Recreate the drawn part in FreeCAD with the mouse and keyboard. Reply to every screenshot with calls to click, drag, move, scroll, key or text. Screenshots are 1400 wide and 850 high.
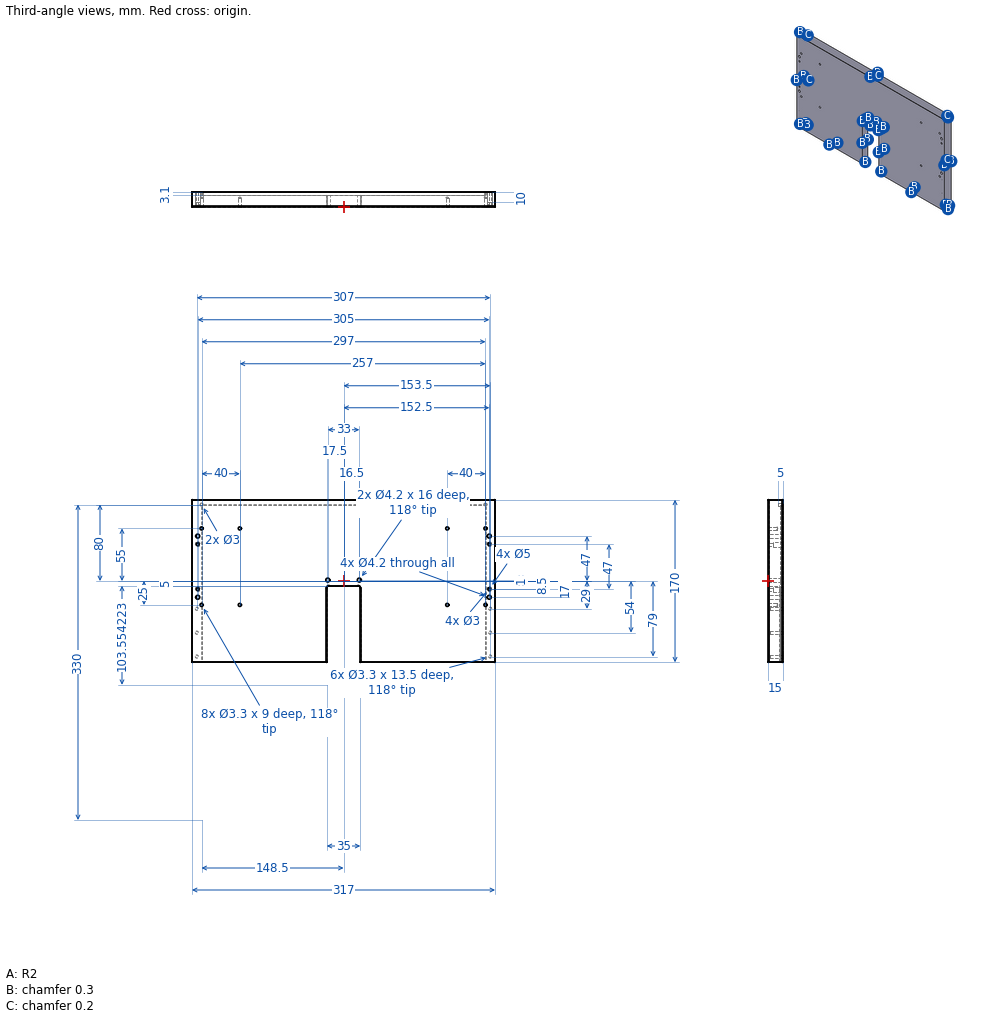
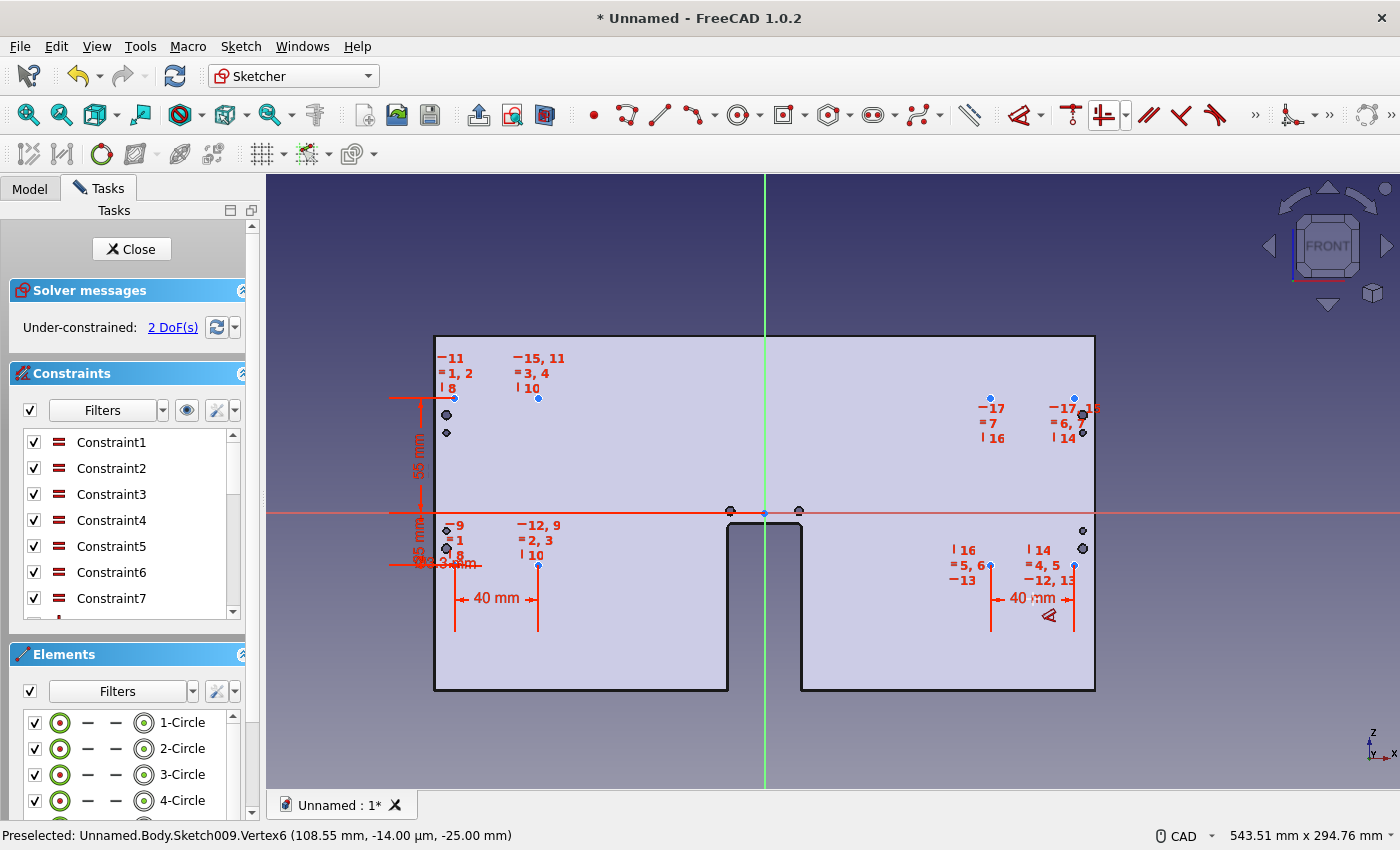
click(538, 565)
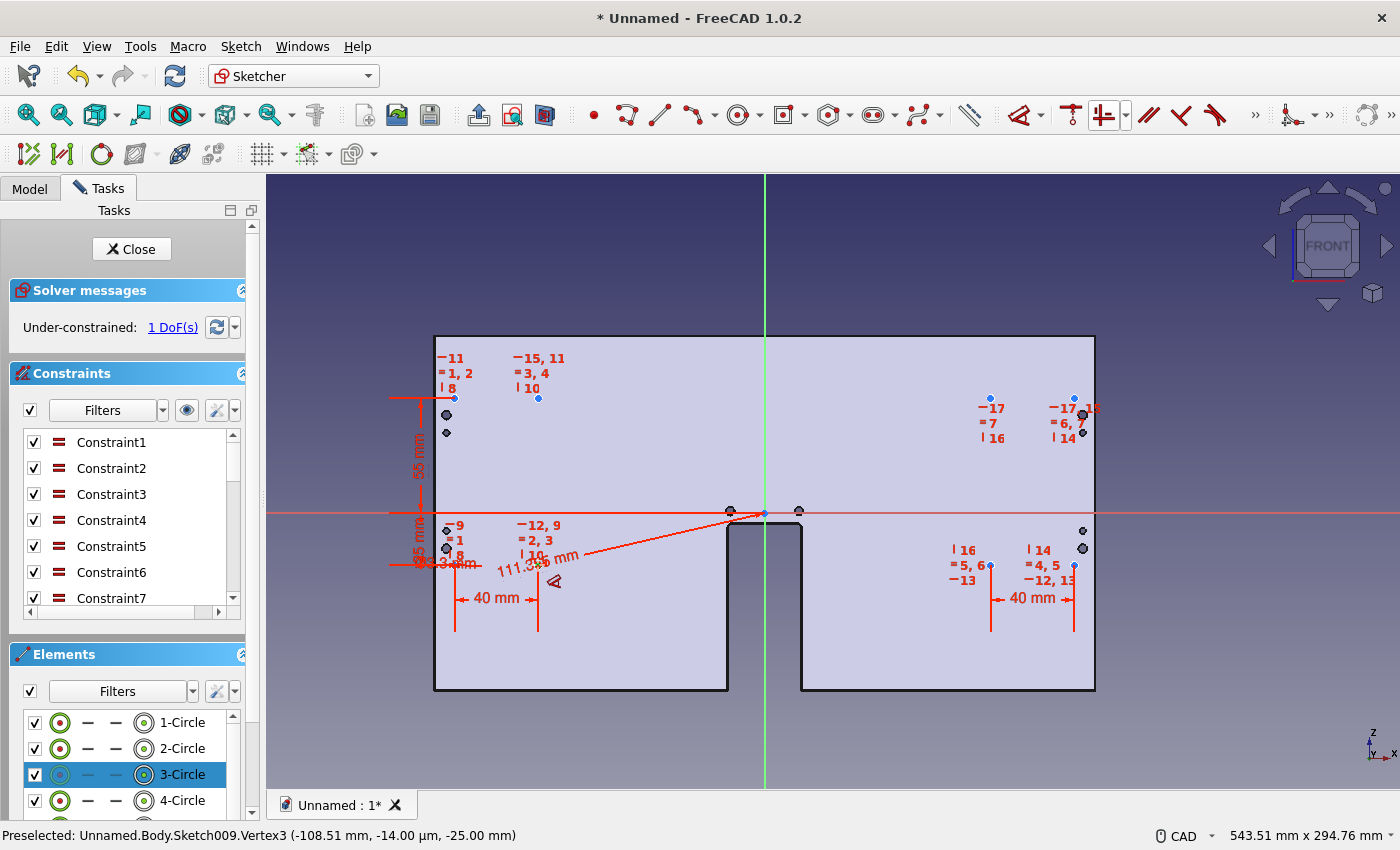
click(1074, 565)
click(806, 599)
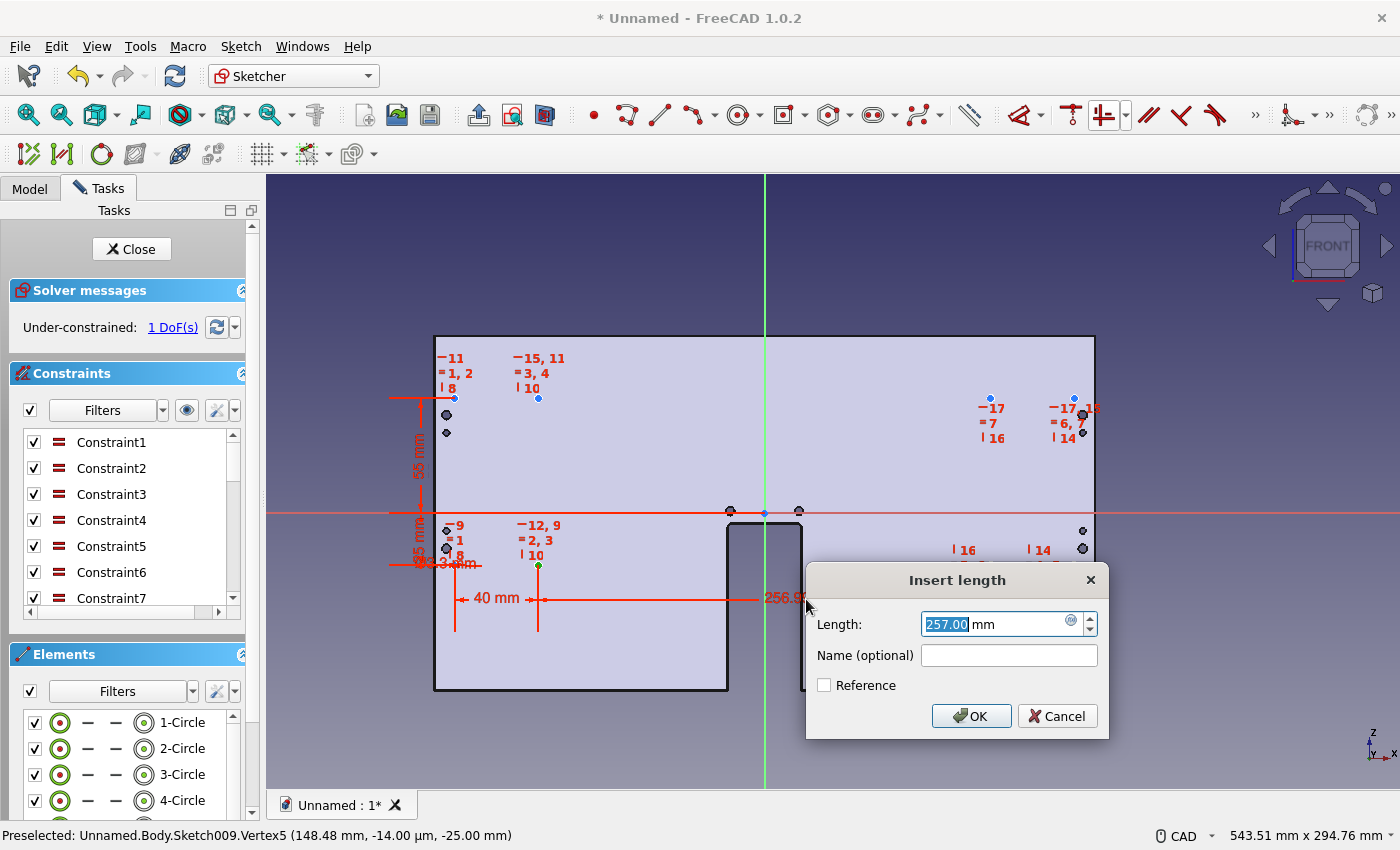
text(257)
key(Return)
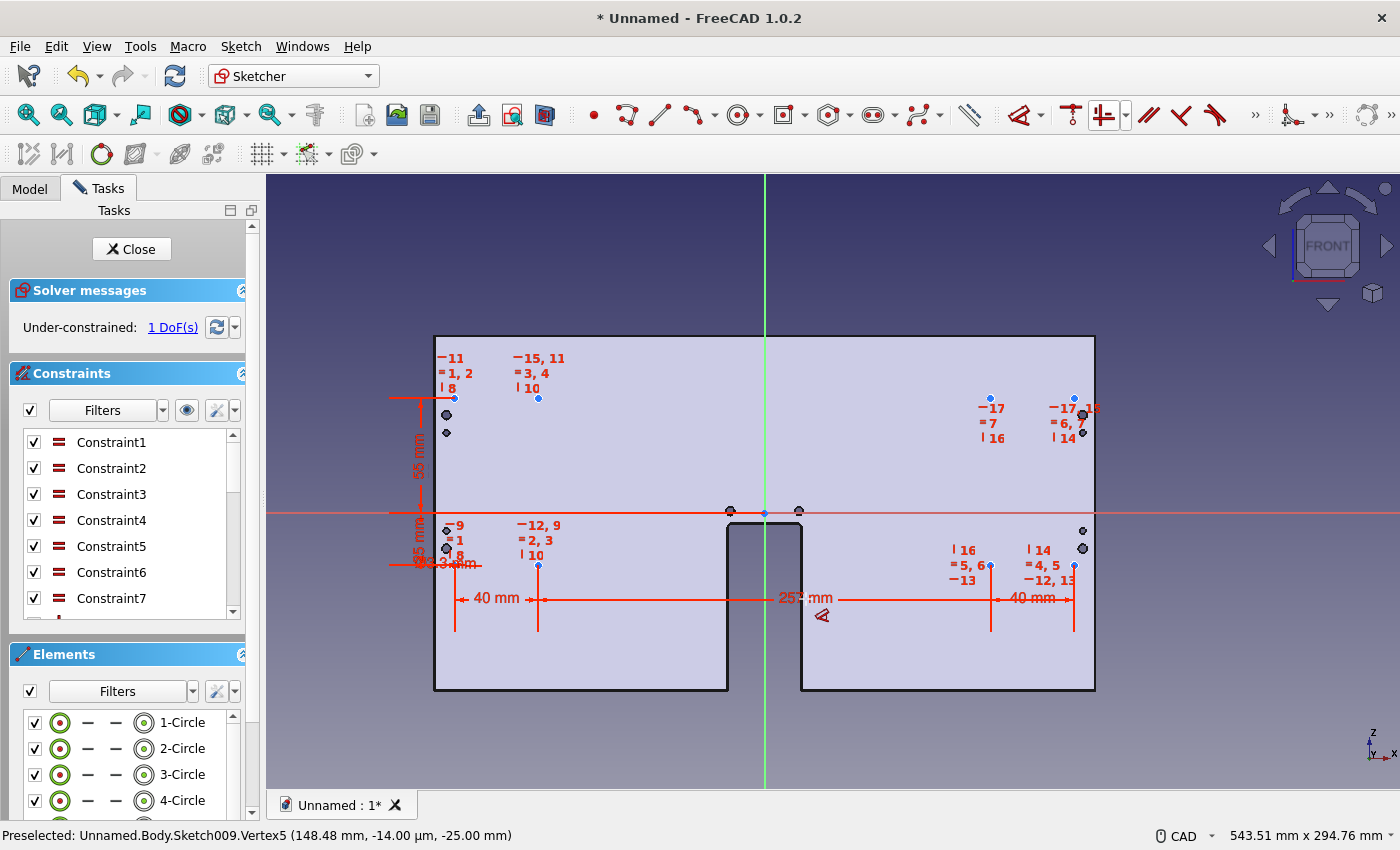
click(455, 565)
click(610, 599)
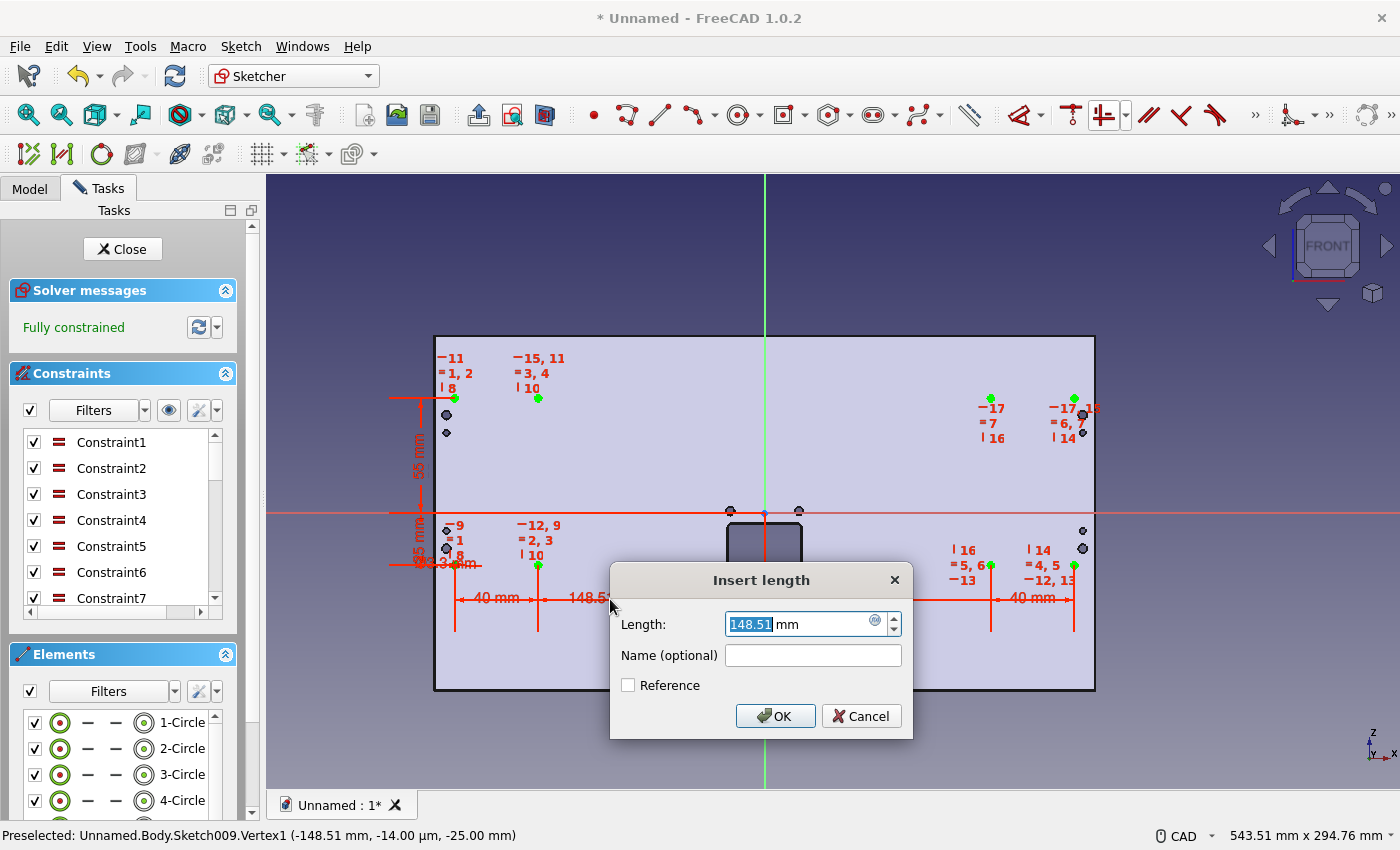
text(148.5)
key(Return)
key(Escape)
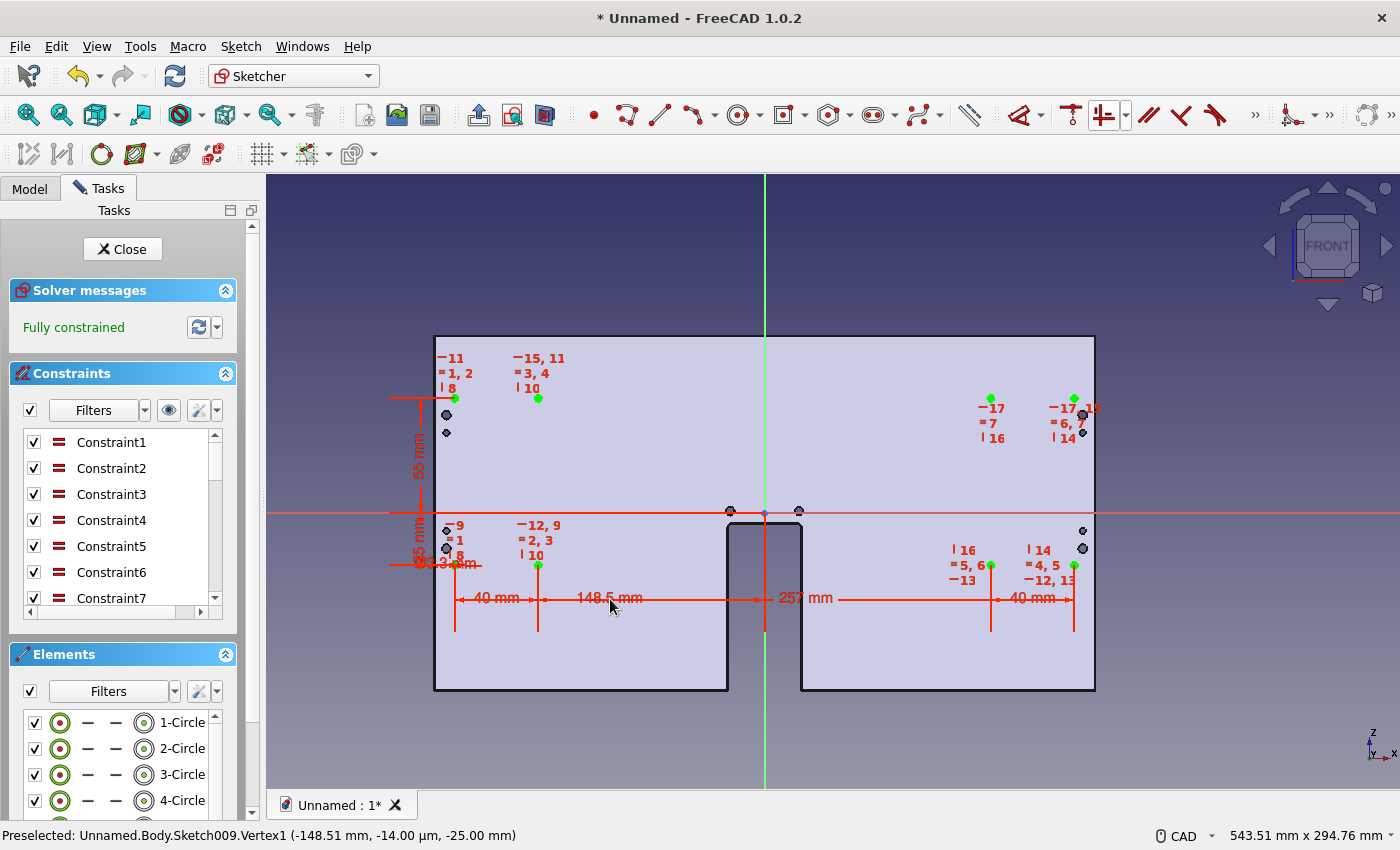
click(123, 249)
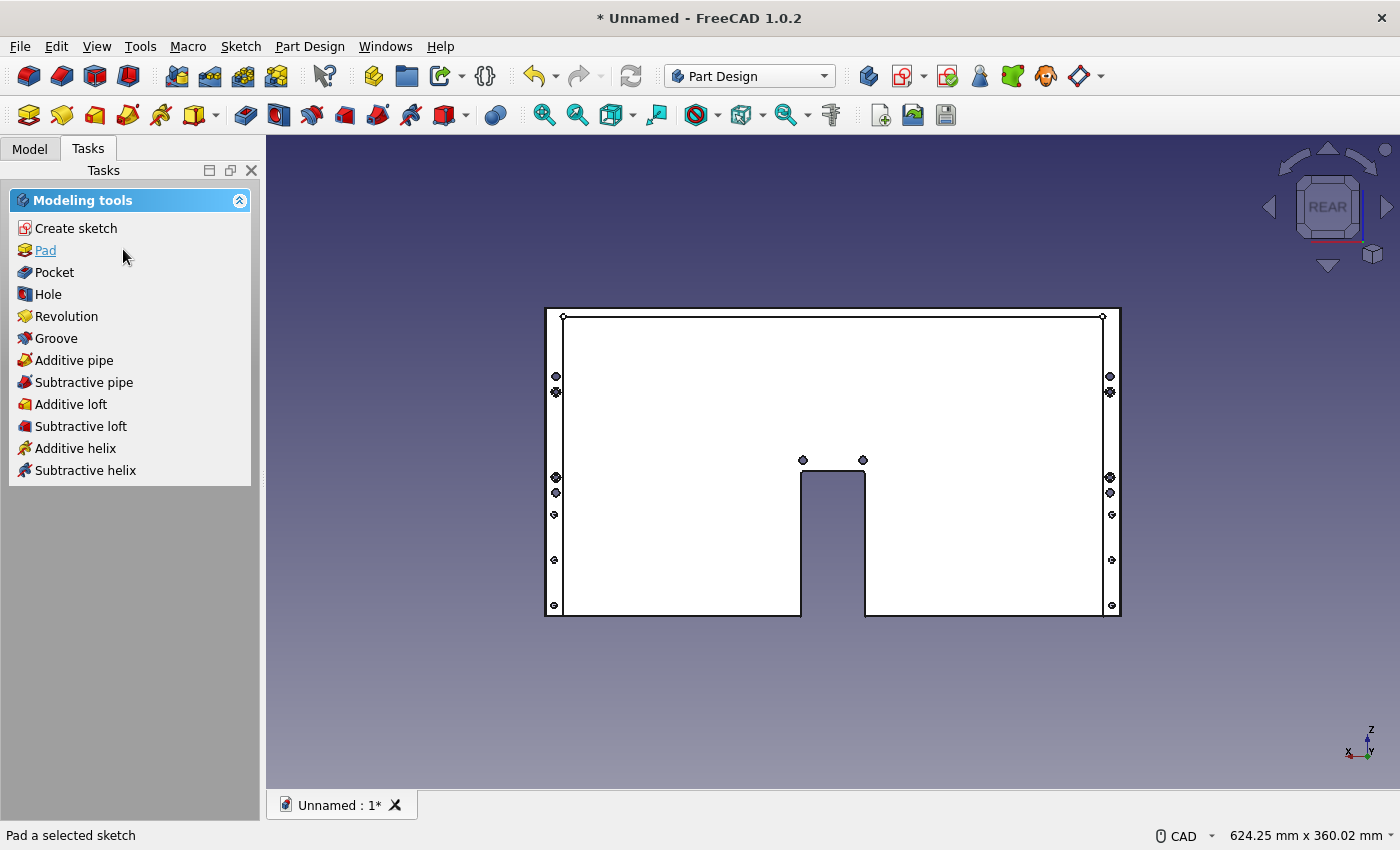
click(279, 116)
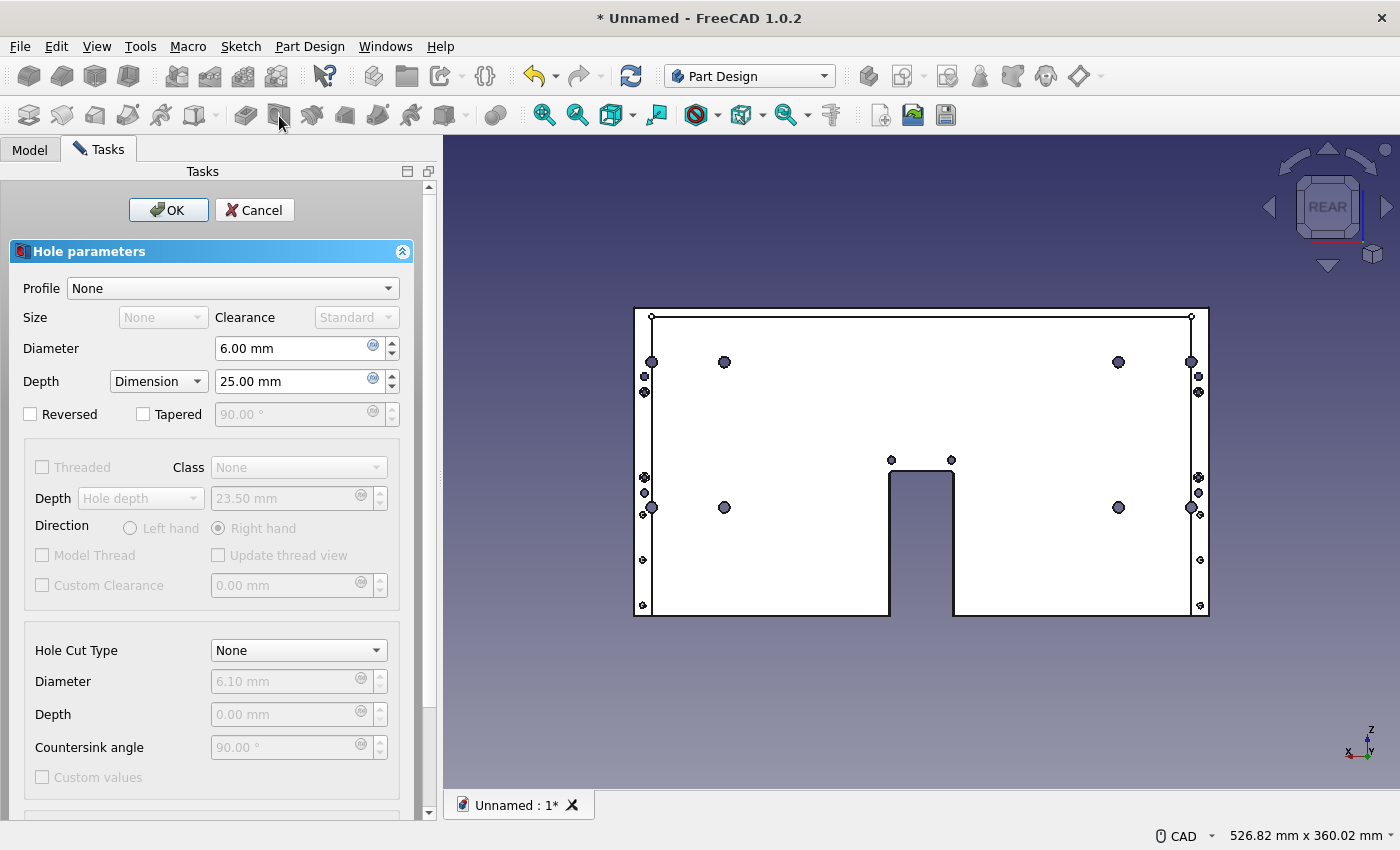
triple_click(300, 348)